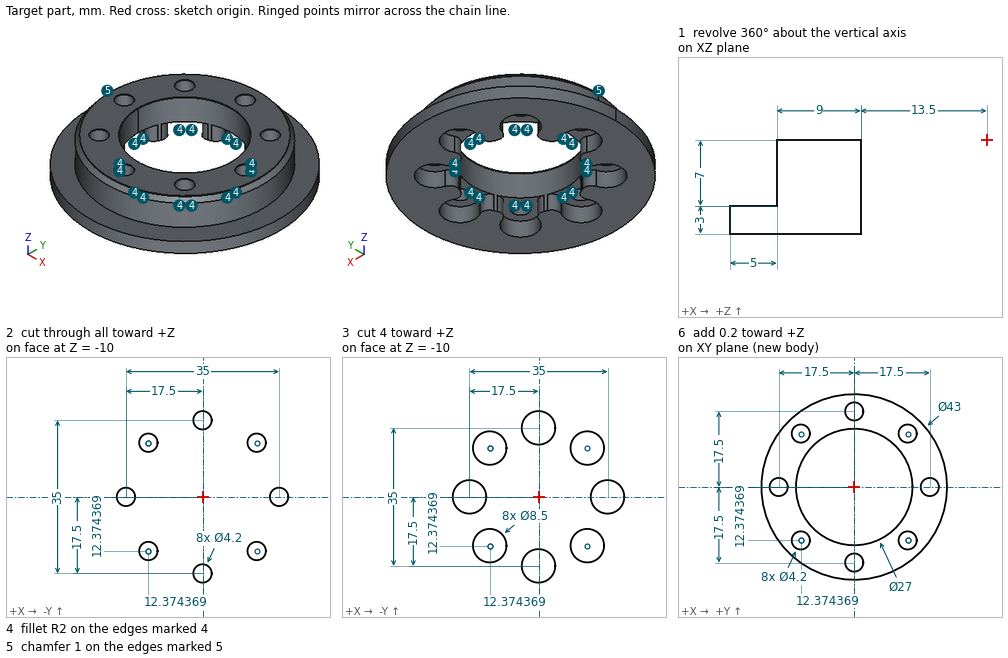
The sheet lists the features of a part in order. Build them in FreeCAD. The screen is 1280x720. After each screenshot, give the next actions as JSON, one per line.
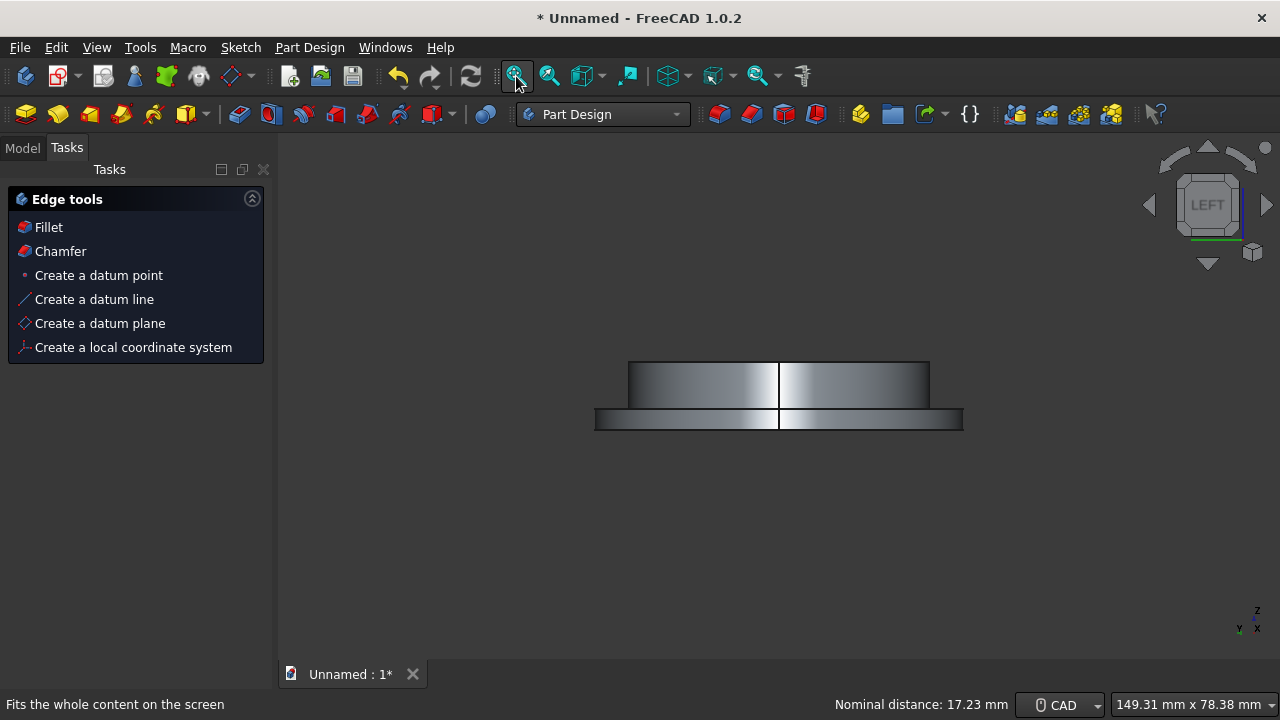
{"action": "key", "text": "0"}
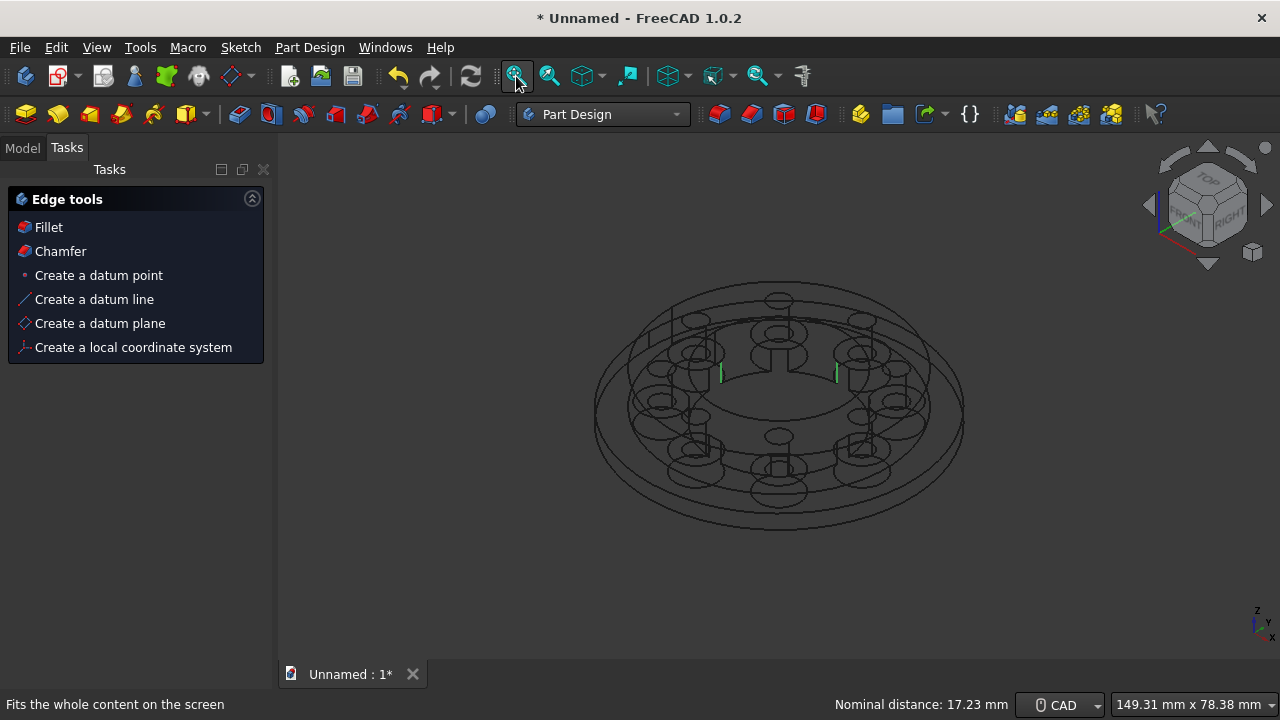
{"action": "left_click", "coordinate": [849, 378], "text": "ctrl"}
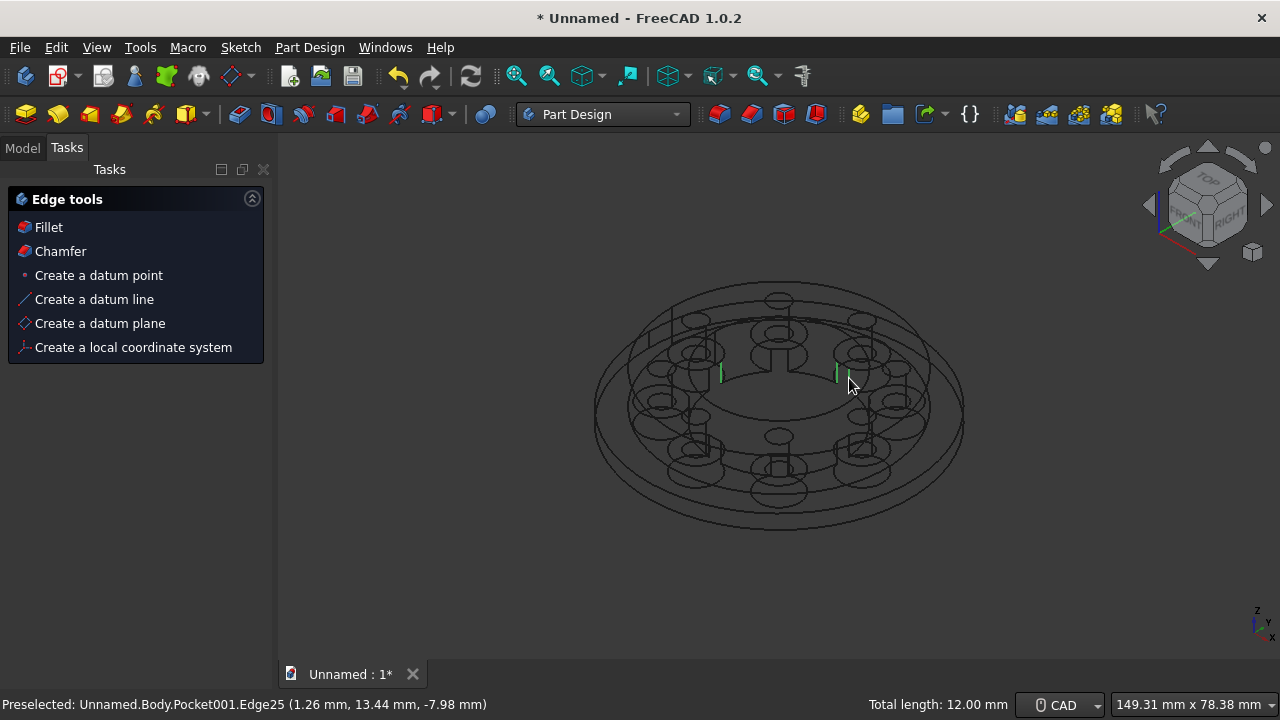
{"action": "left_click", "coordinate": [788, 359], "text": "ctrl"}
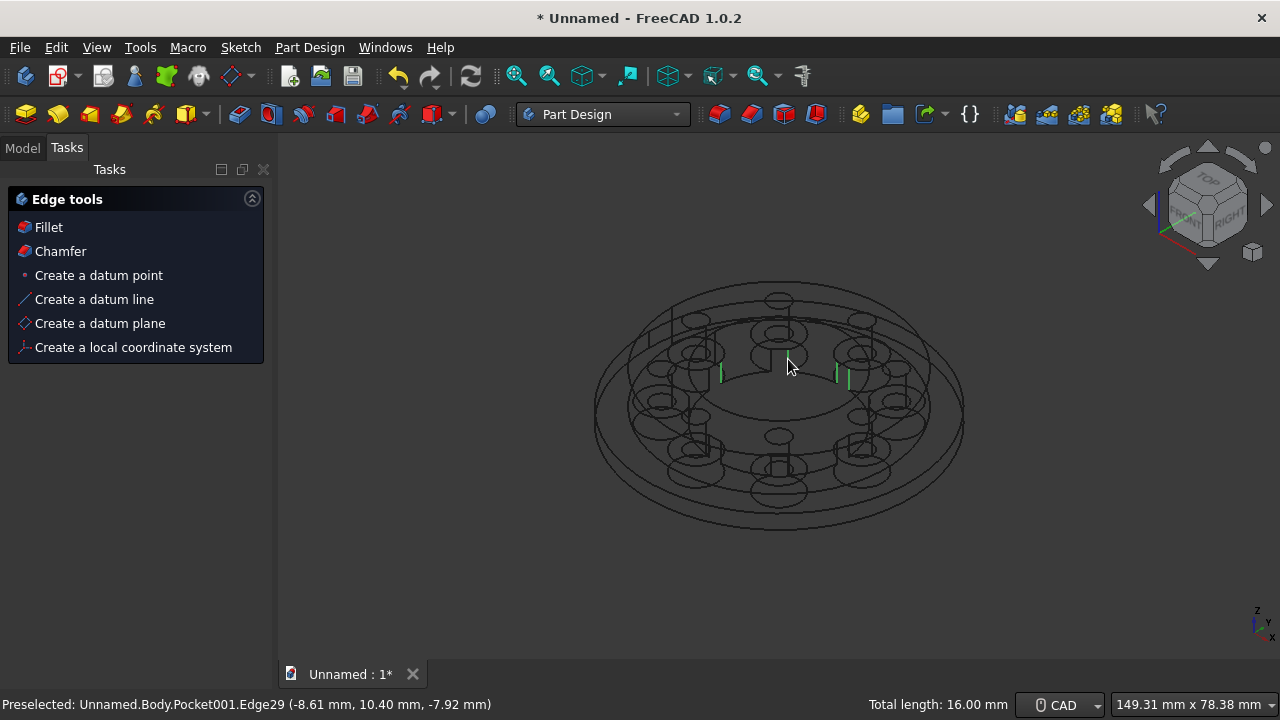
{"action": "left_click", "coordinate": [771, 359], "text": "ctrl"}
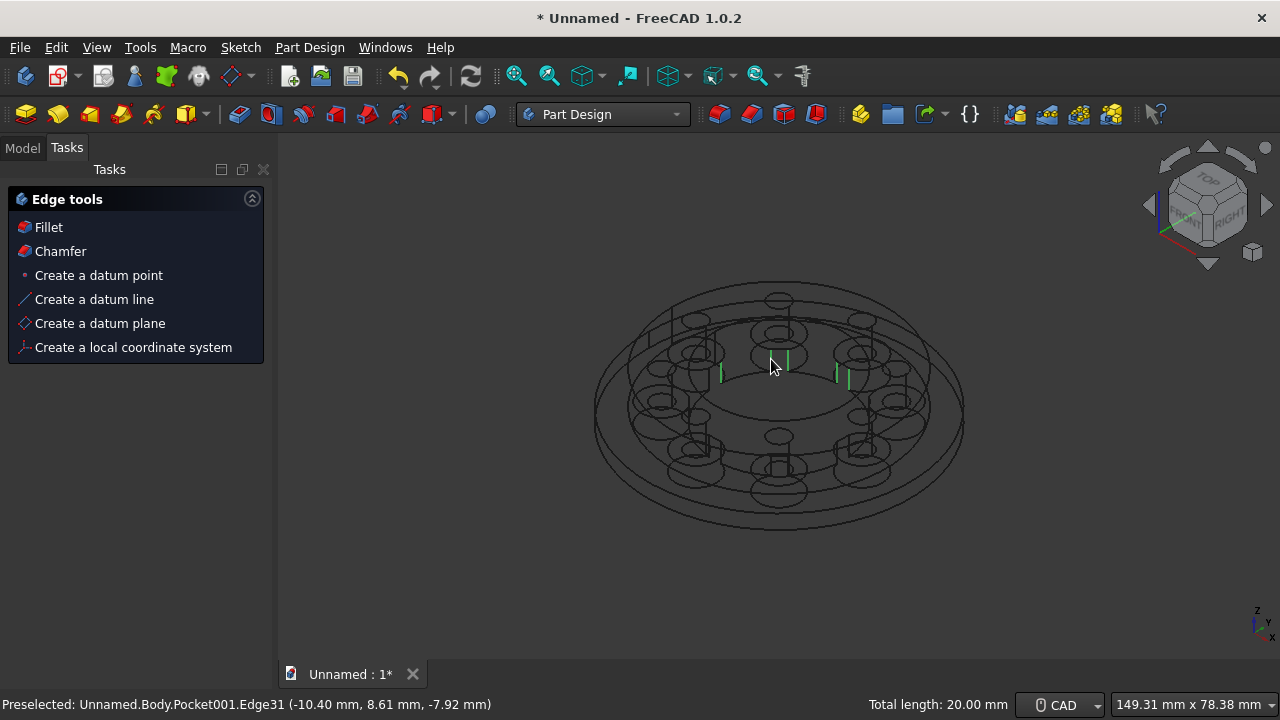
{"action": "left_click", "coordinate": [709, 378], "text": "ctrl"}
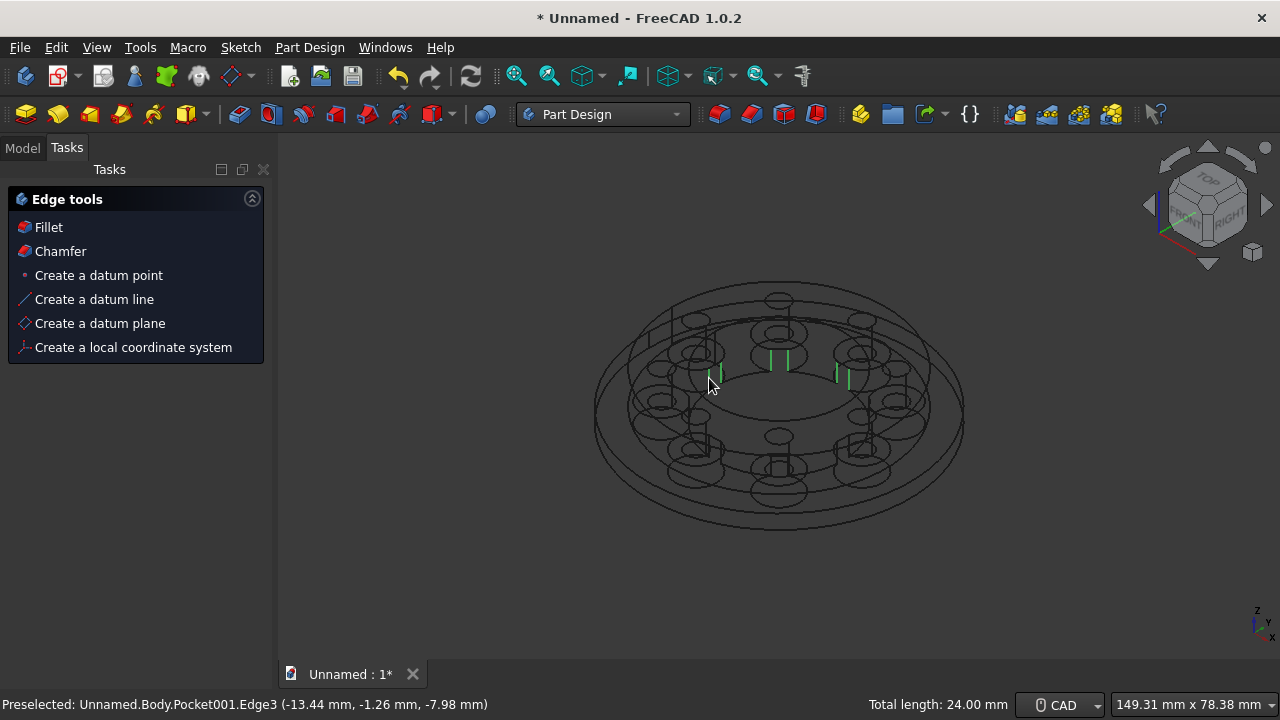
{"action": "key", "text": "2"}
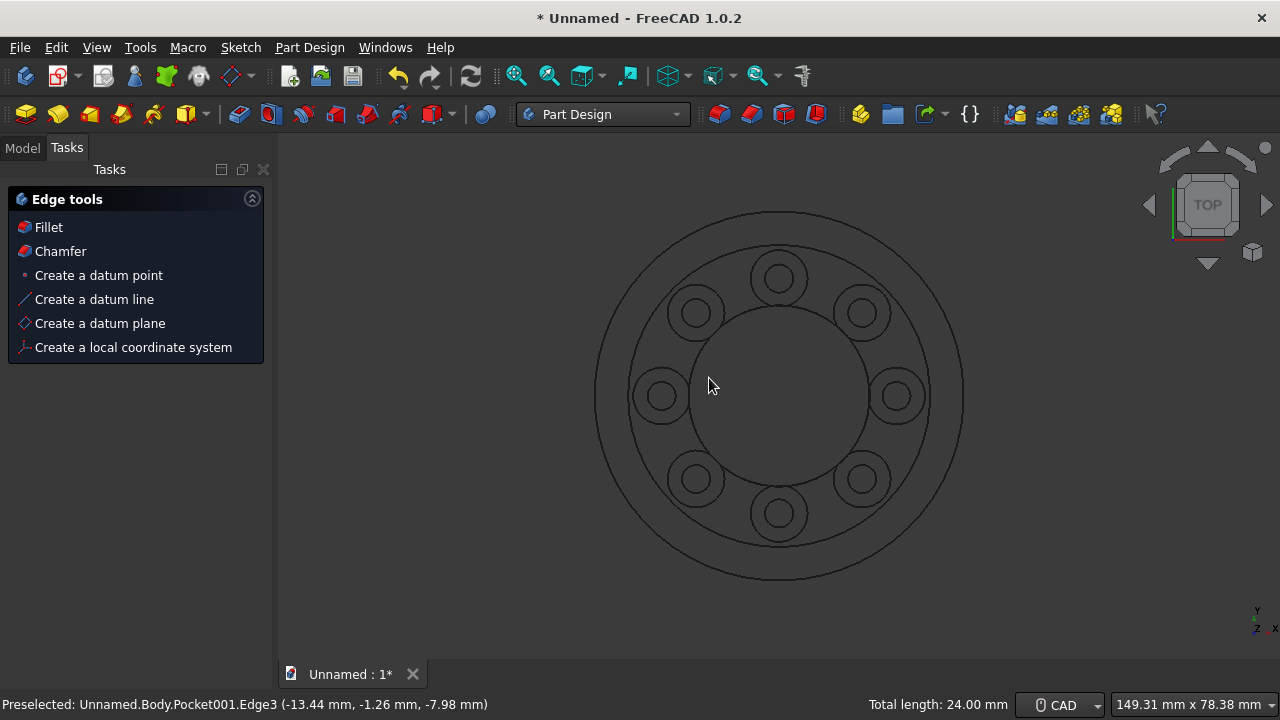
{"action": "key", "text": "1"}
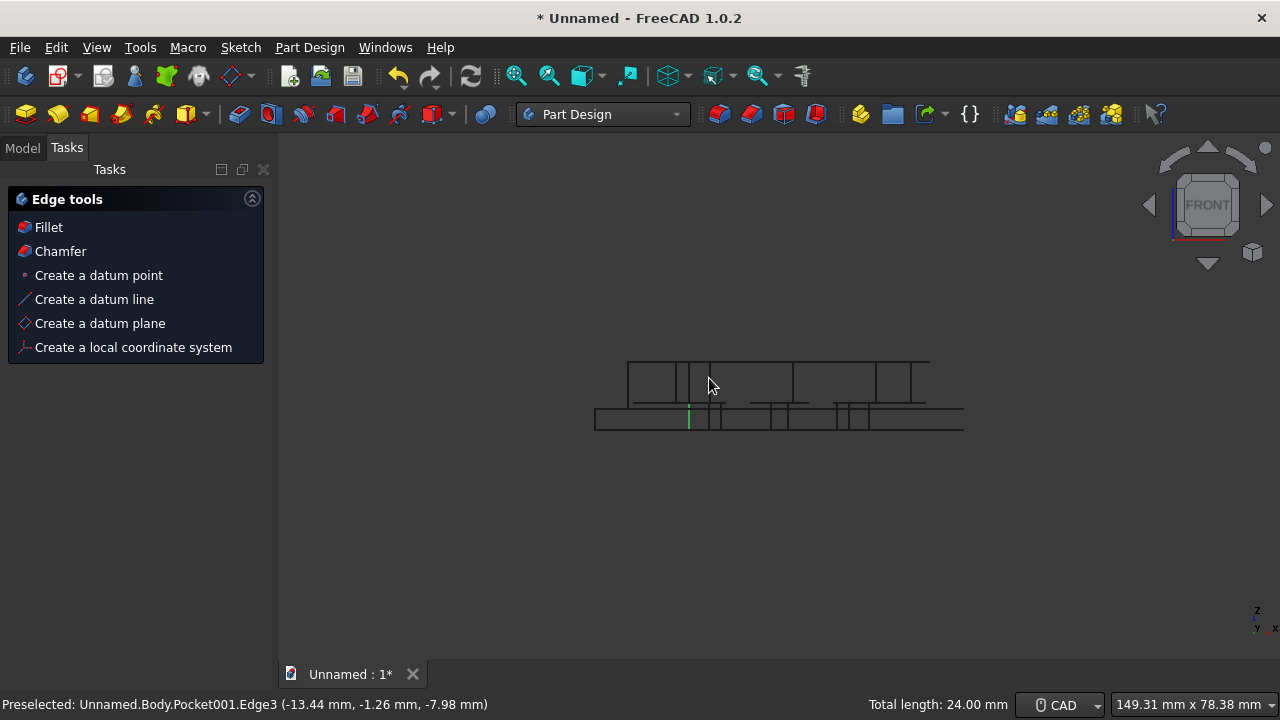
{"action": "key", "text": "v f"}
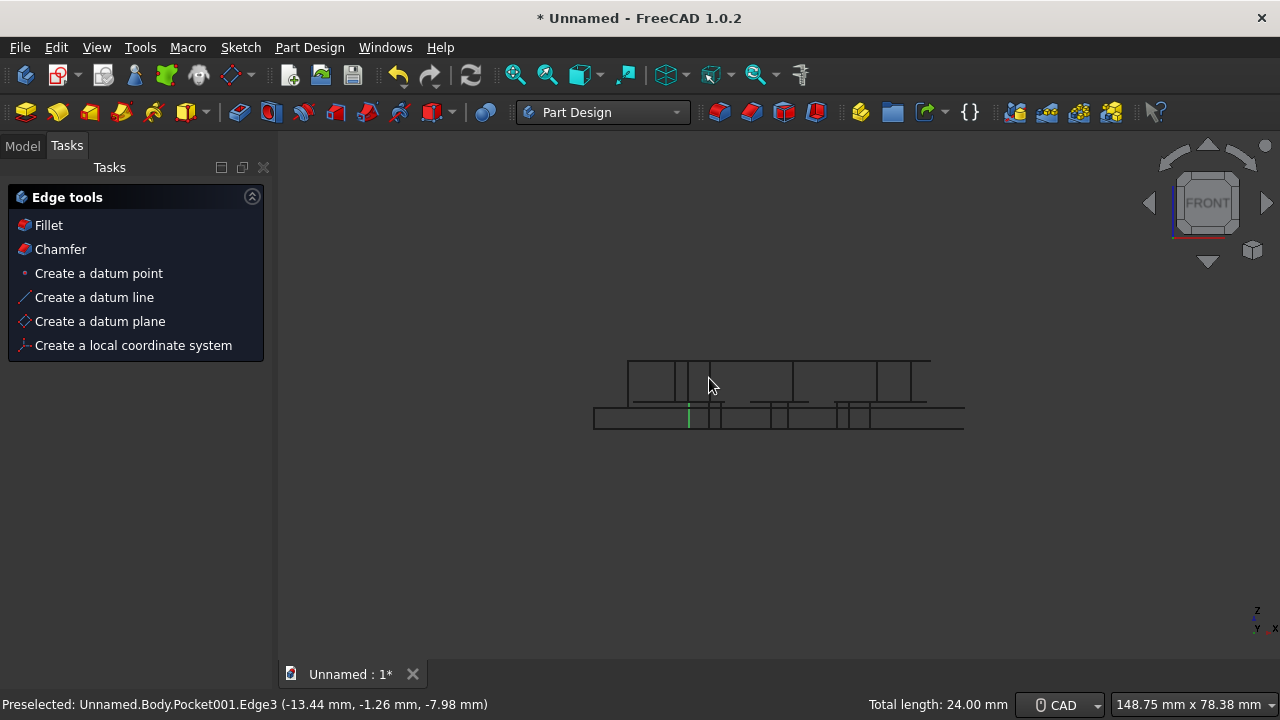
{"action": "left_click", "coordinate": [709, 414], "text": "ctrl"}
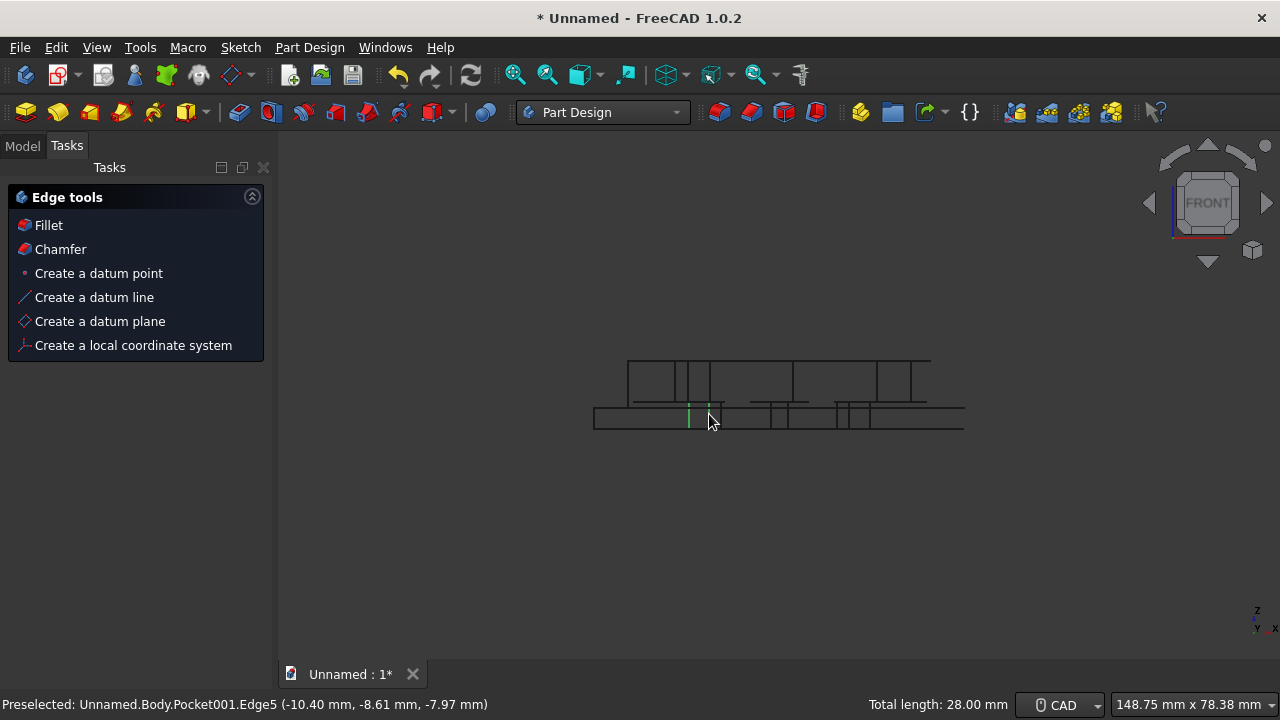
{"action": "left_click", "coordinate": [721, 414], "text": "ctrl"}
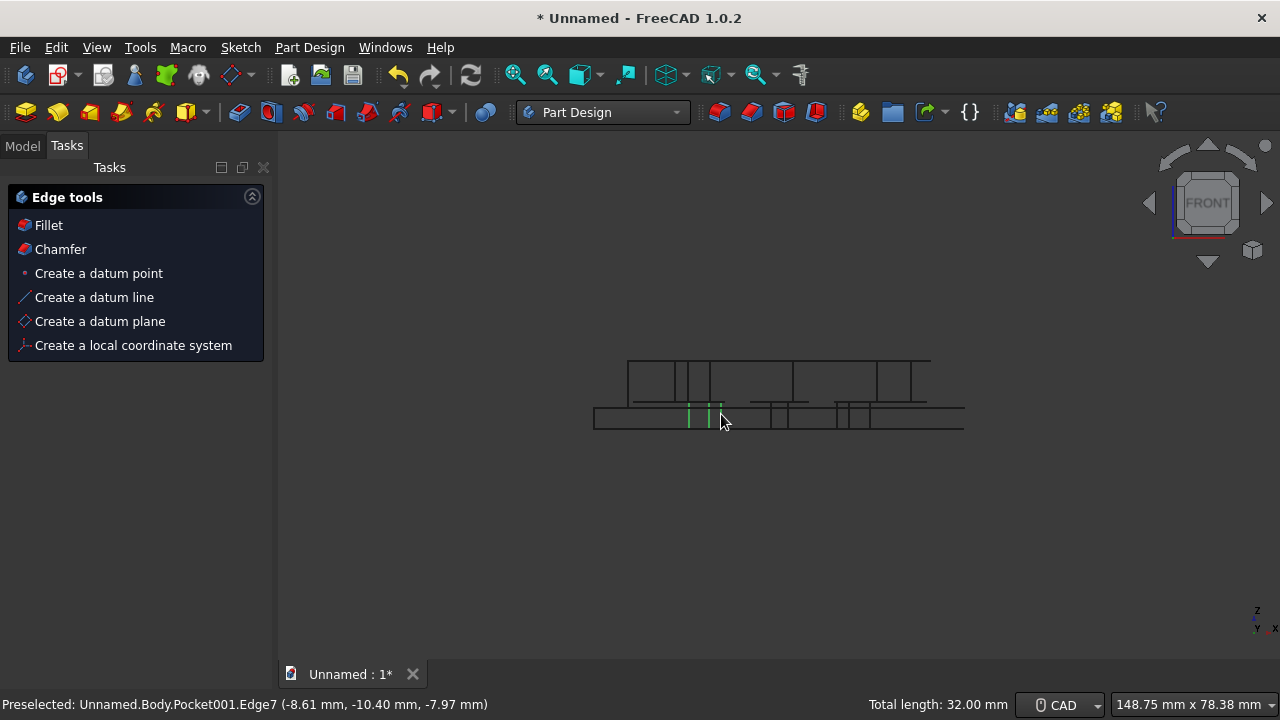
{"action": "left_click", "coordinate": [771, 414], "text": "ctrl"}